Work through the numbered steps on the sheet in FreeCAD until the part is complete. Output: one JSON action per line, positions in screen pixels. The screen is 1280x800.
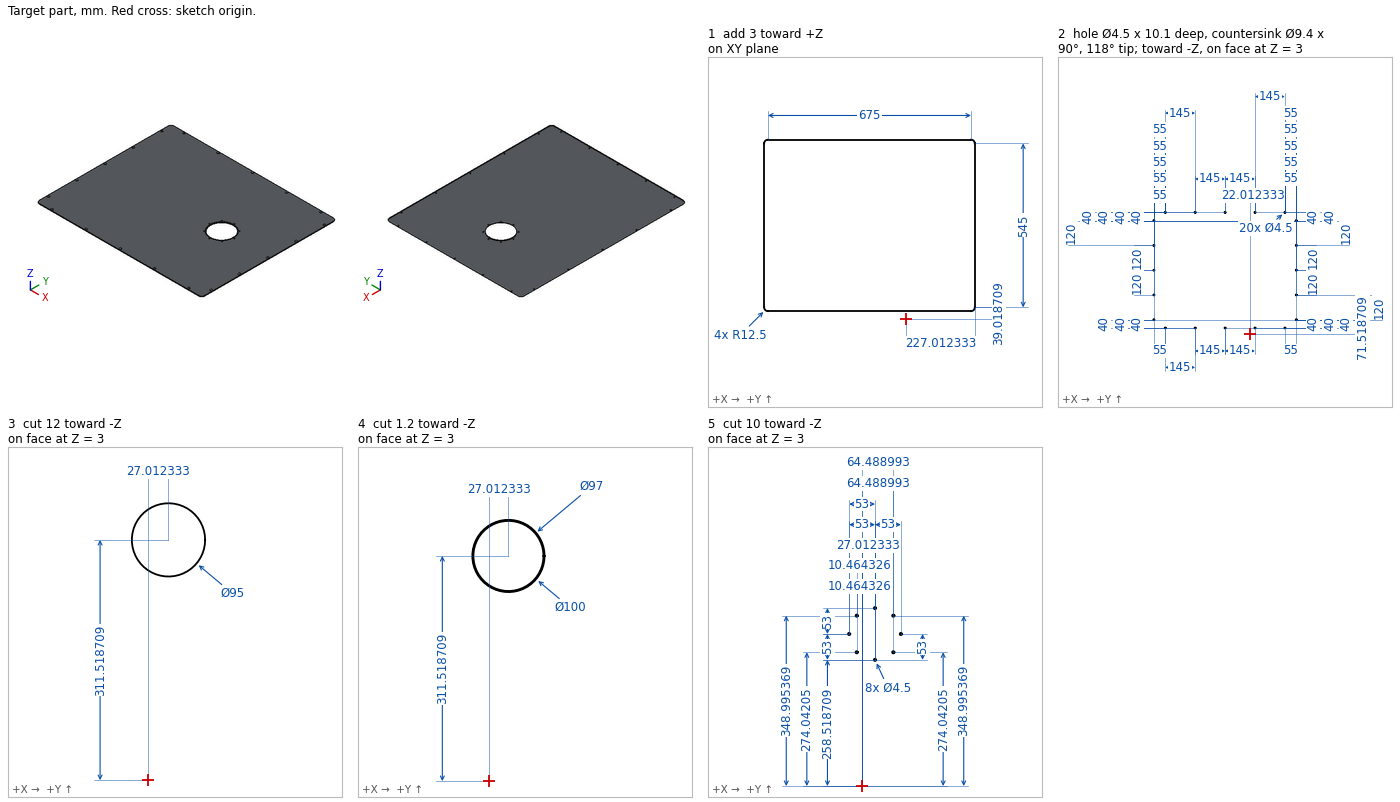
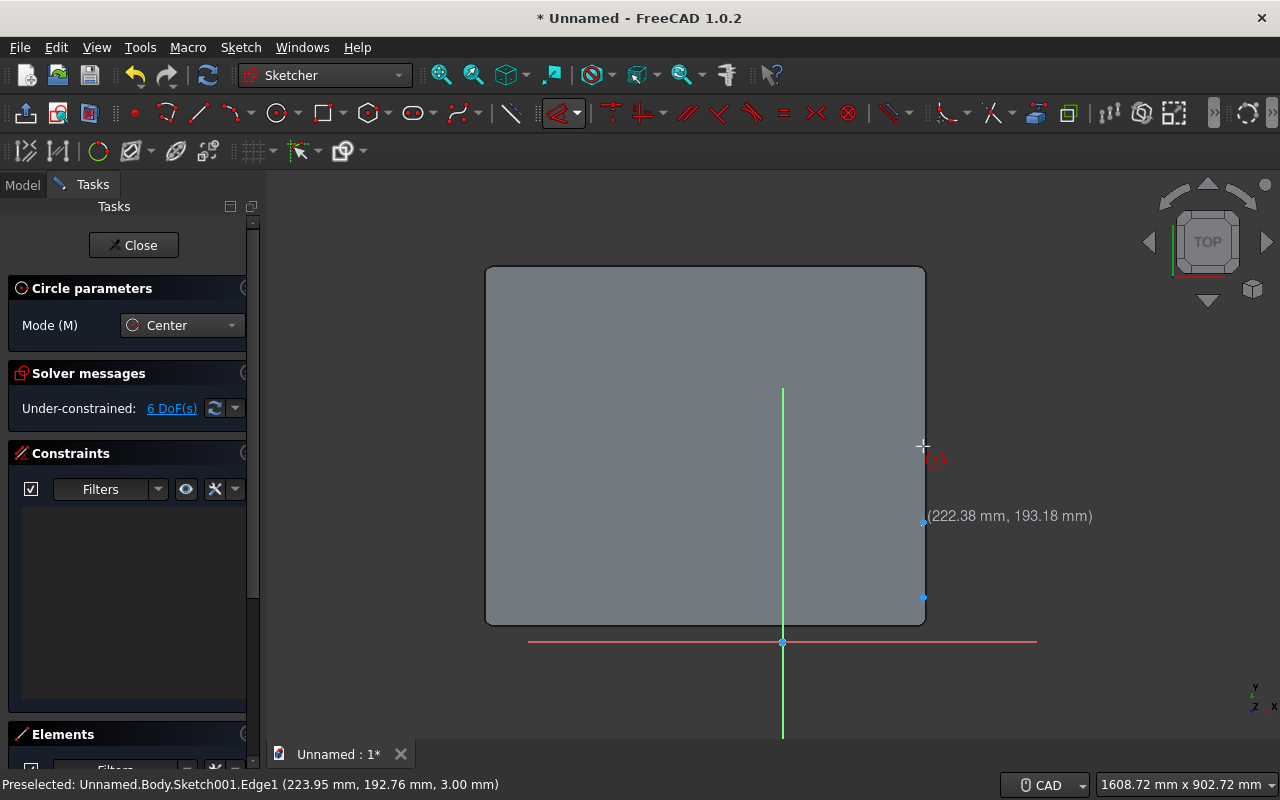
{"action": "left_click", "coordinate": [923, 446]}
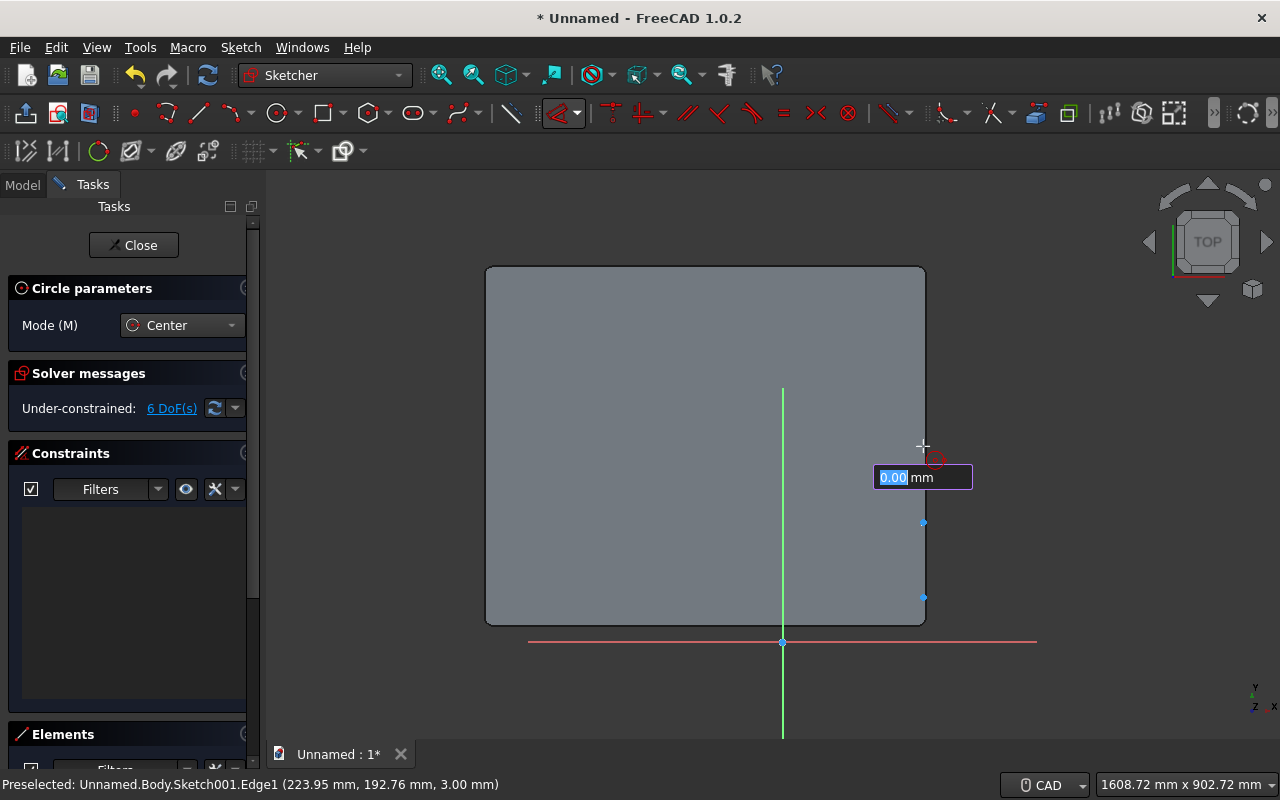
{"action": "scroll", "coordinate": [924, 445], "scroll_direction": "up", "scroll_amount": 13}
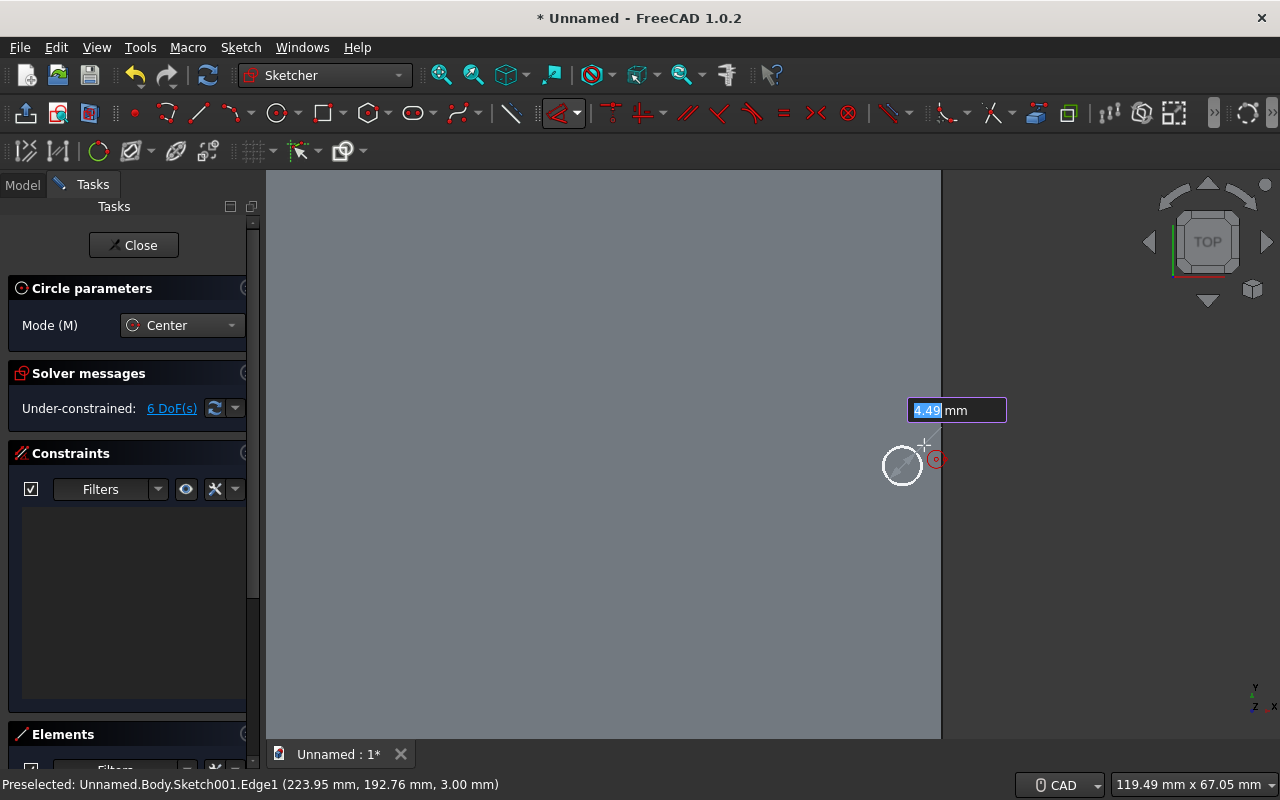
{"action": "left_click", "coordinate": [913, 439]}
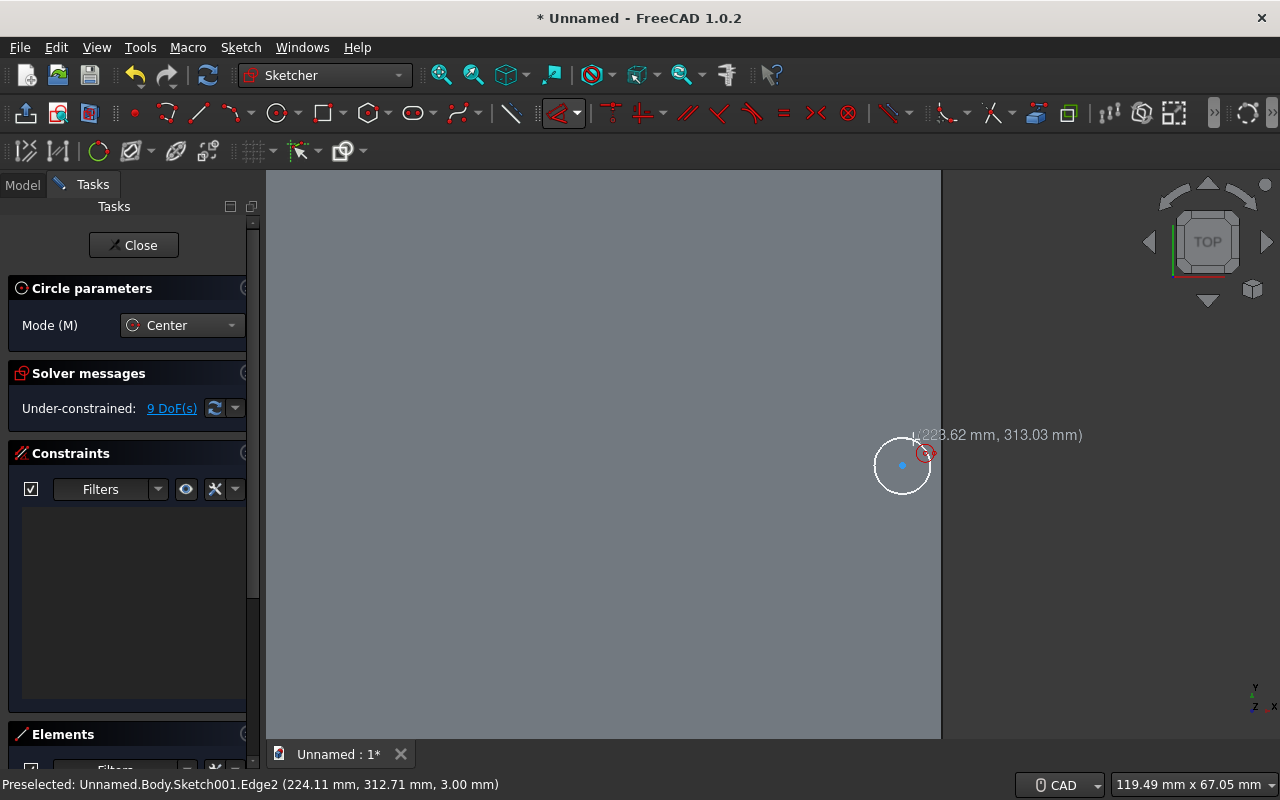
{"action": "scroll", "coordinate": [924, 445], "scroll_direction": "down", "scroll_amount": 13}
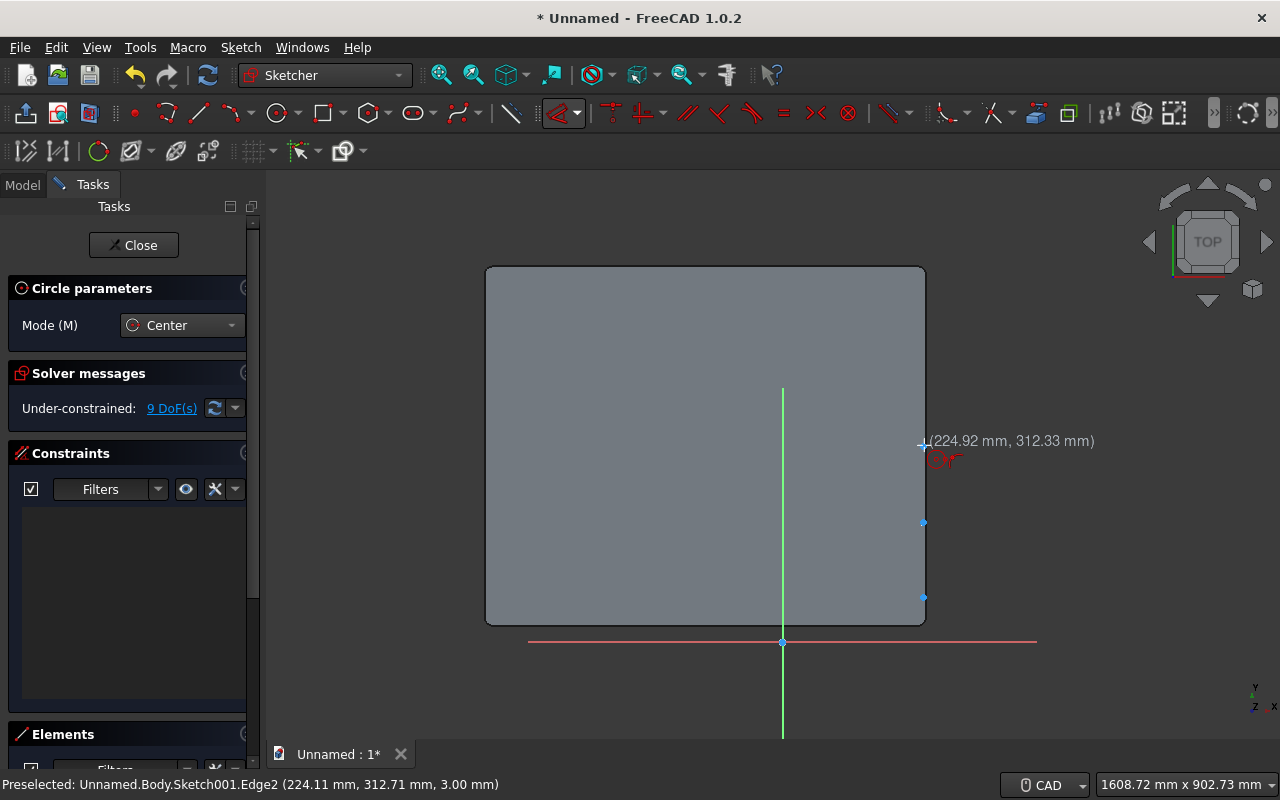
{"action": "scroll", "coordinate": [923, 370], "scroll_direction": "up", "scroll_amount": 14}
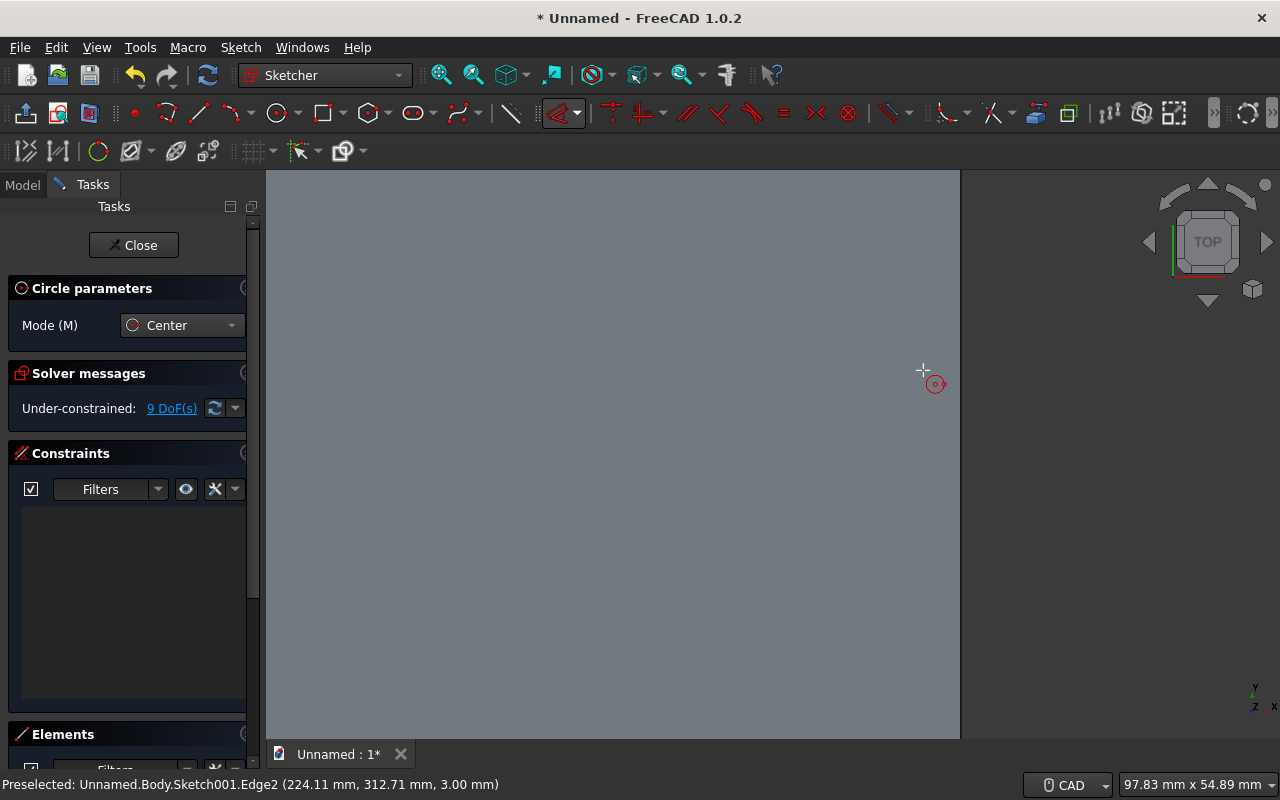
{"action": "scroll", "coordinate": [923, 370], "scroll_direction": "down", "scroll_amount": 14}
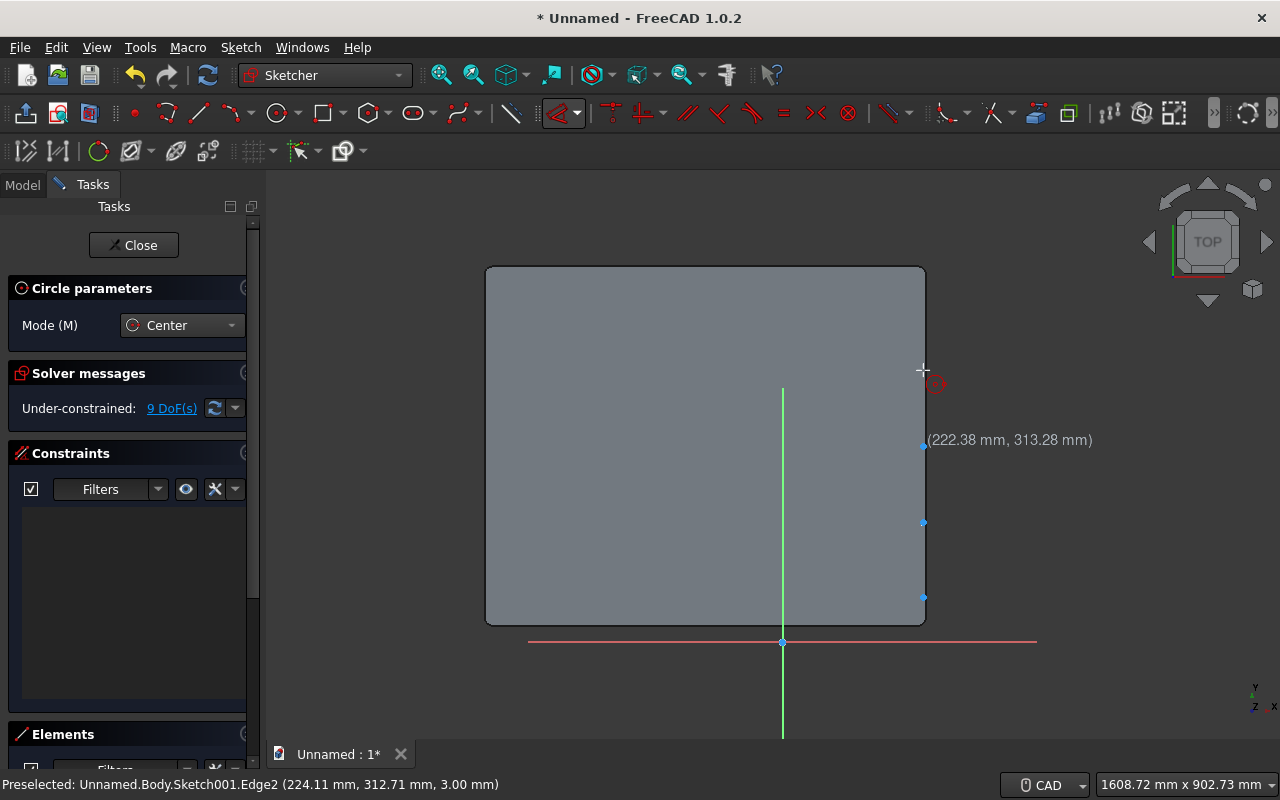
{"action": "left_click", "coordinate": [923, 370]}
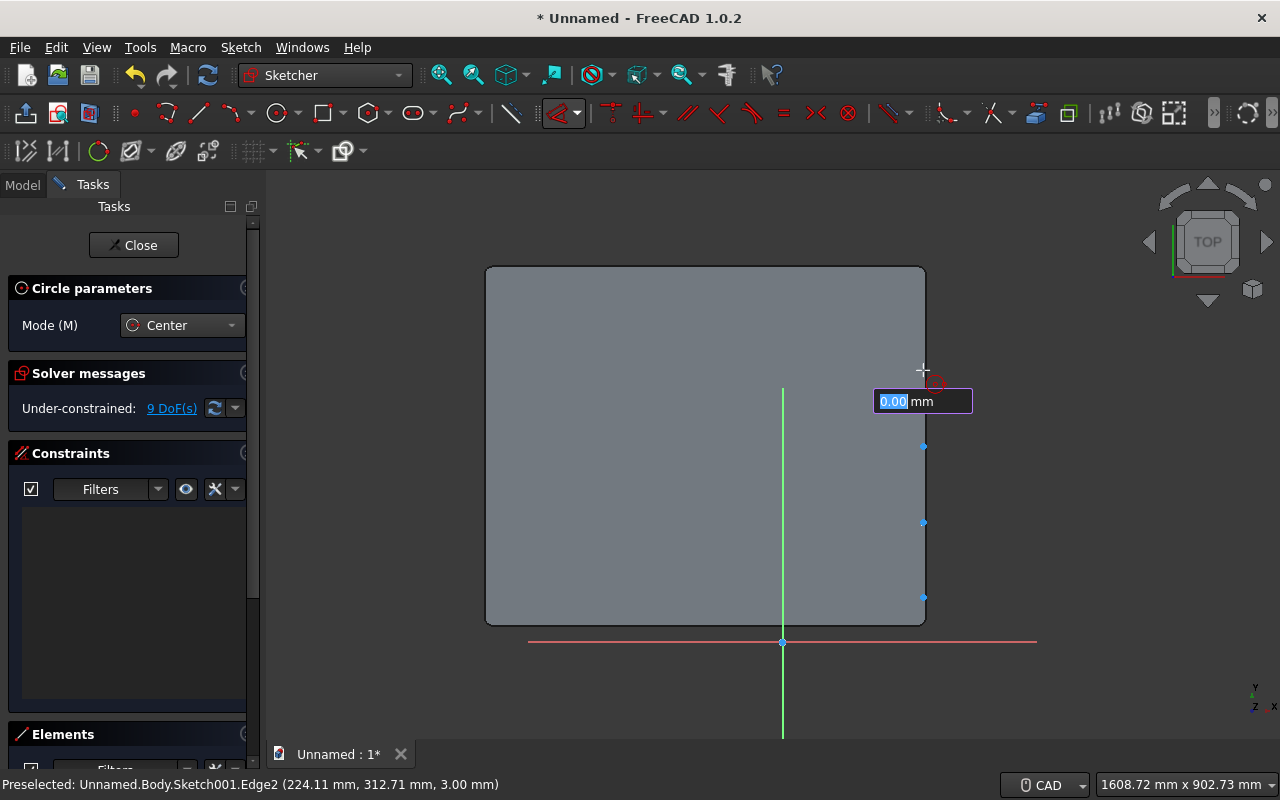
{"action": "scroll", "coordinate": [924, 369], "scroll_direction": "up", "scroll_amount": 13}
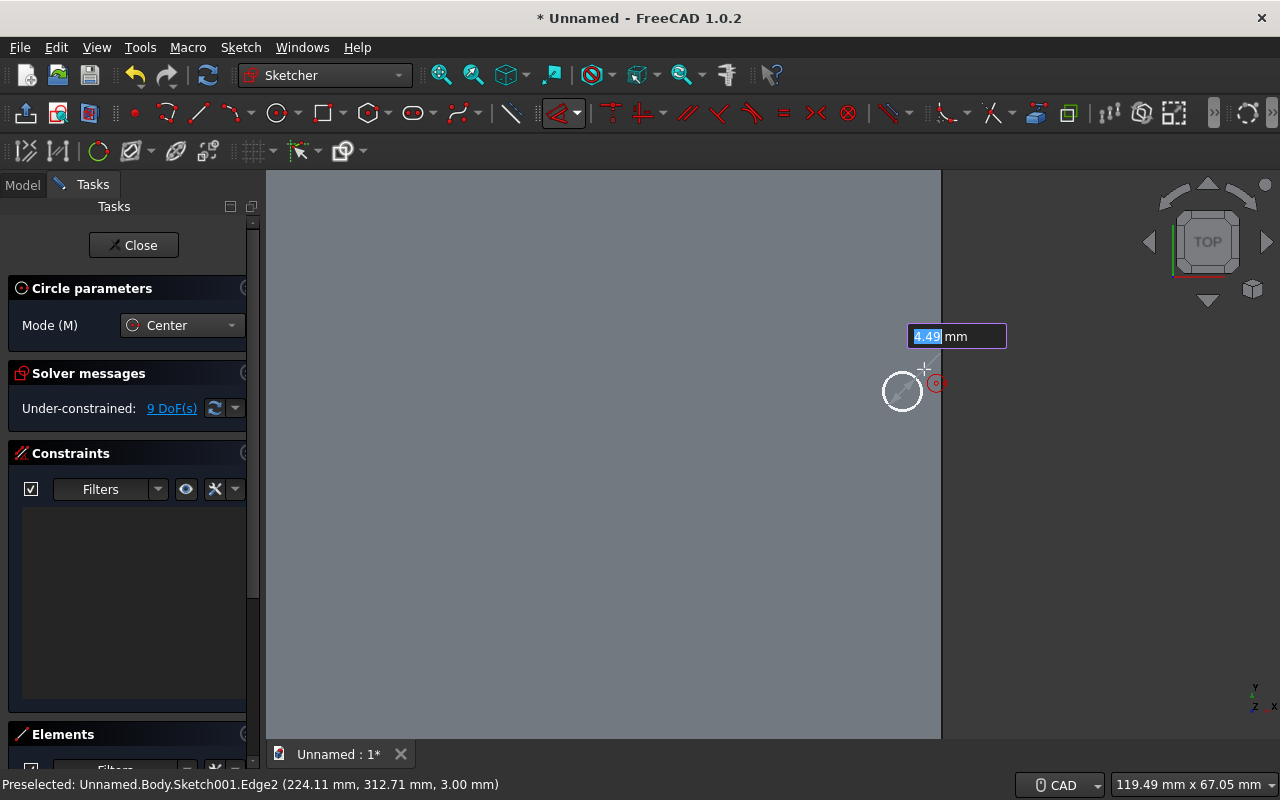
{"action": "left_click", "coordinate": [913, 370]}